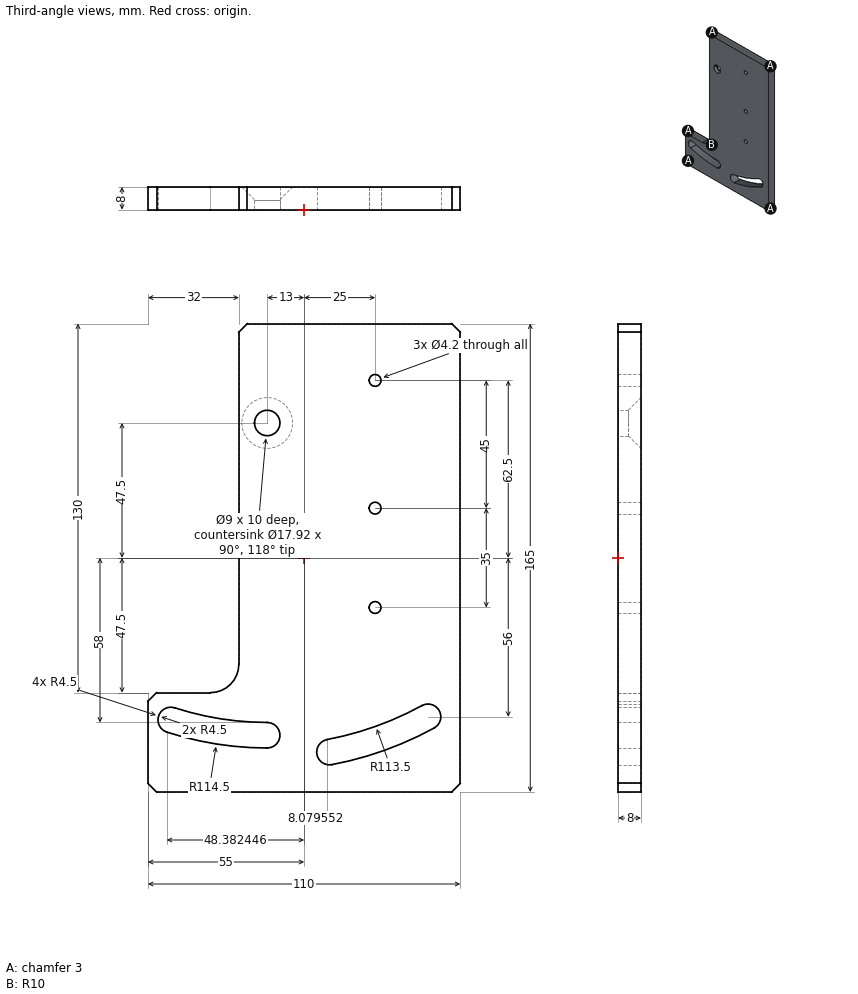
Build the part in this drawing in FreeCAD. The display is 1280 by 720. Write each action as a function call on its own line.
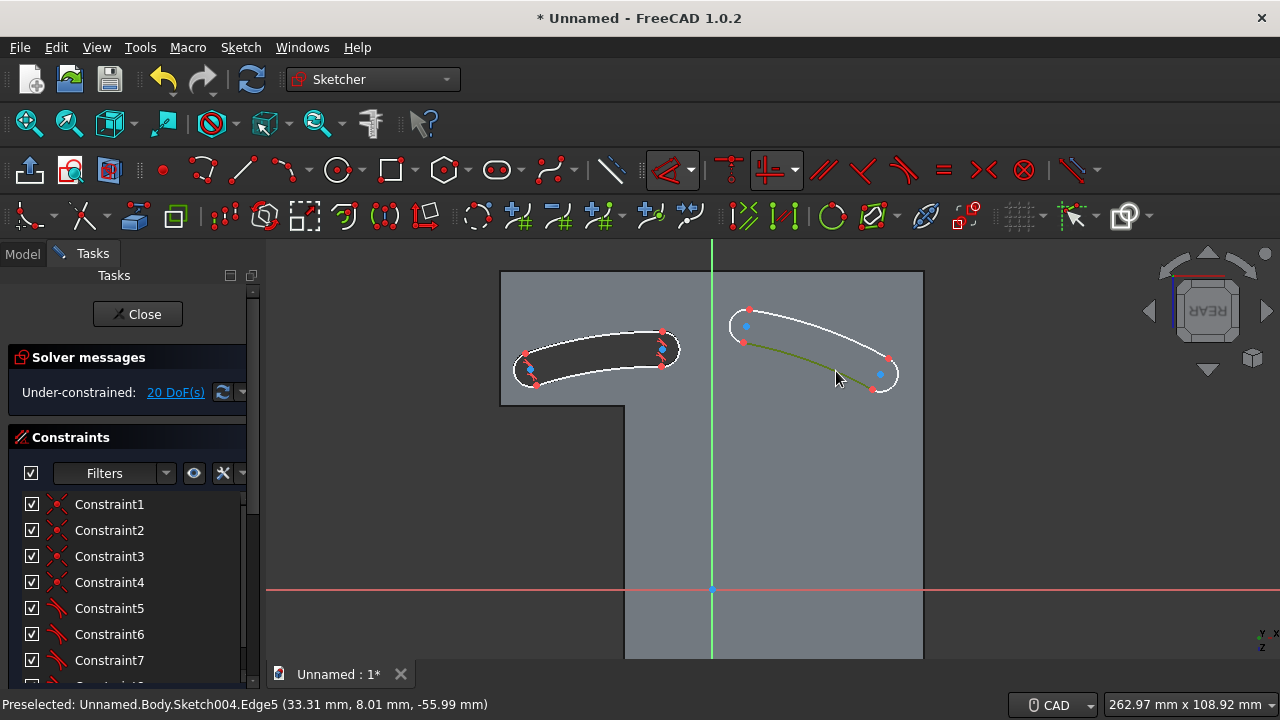
click(888, 390)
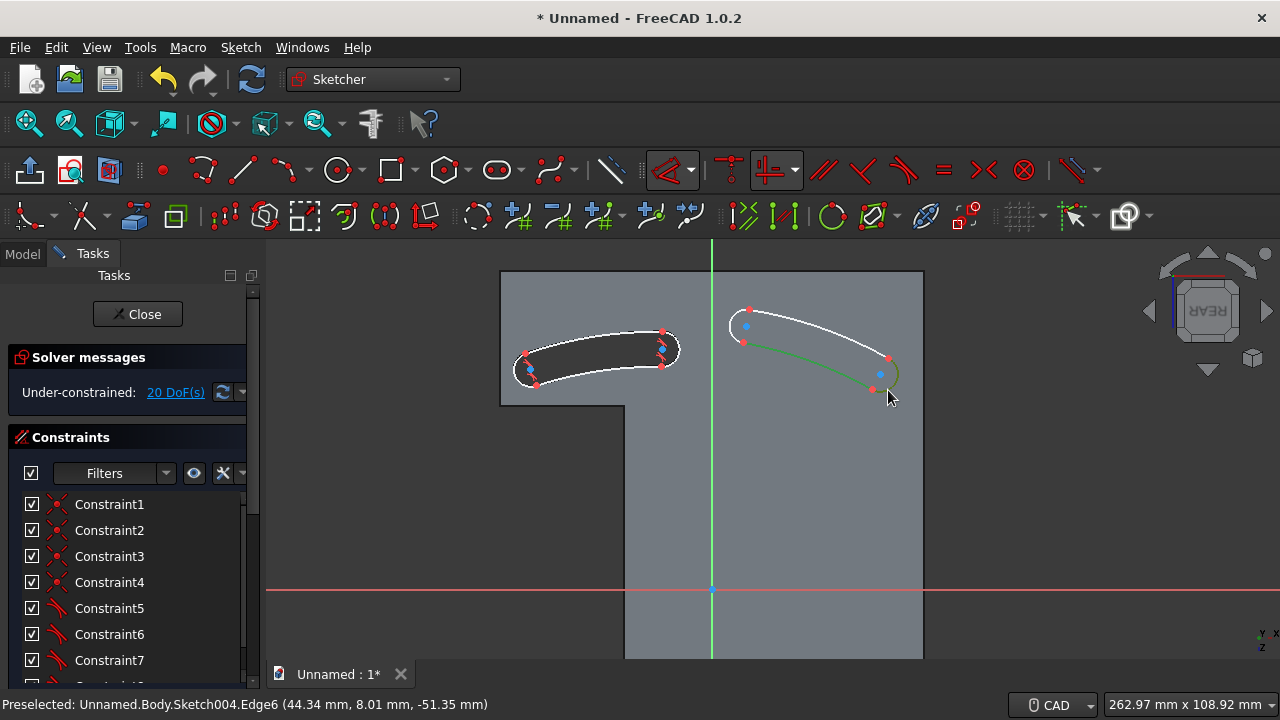
click(904, 170)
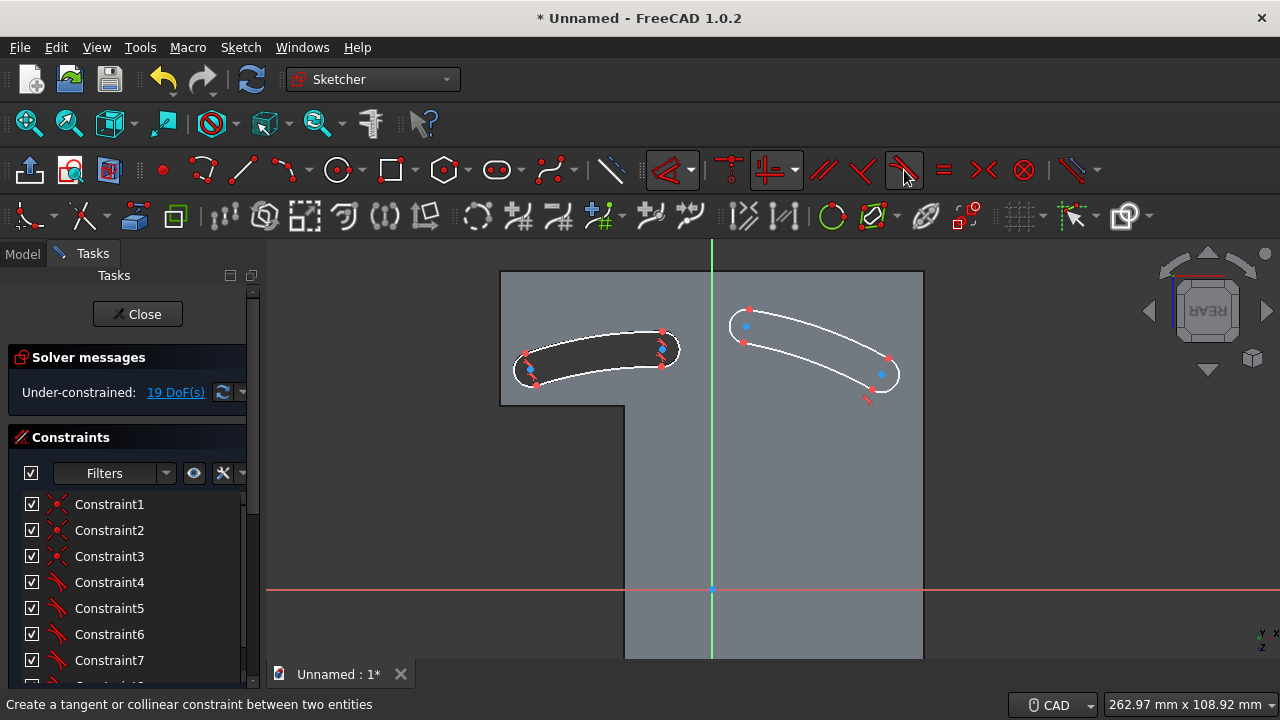
click(836, 371)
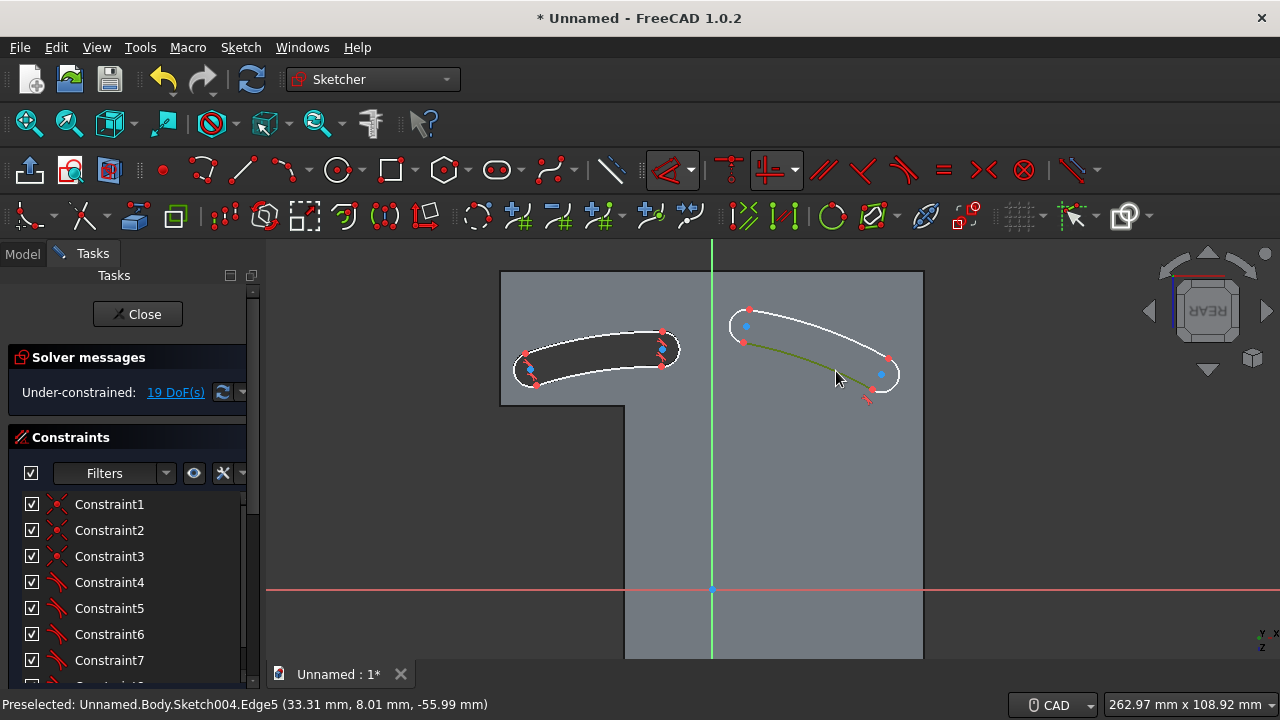
click(735, 314)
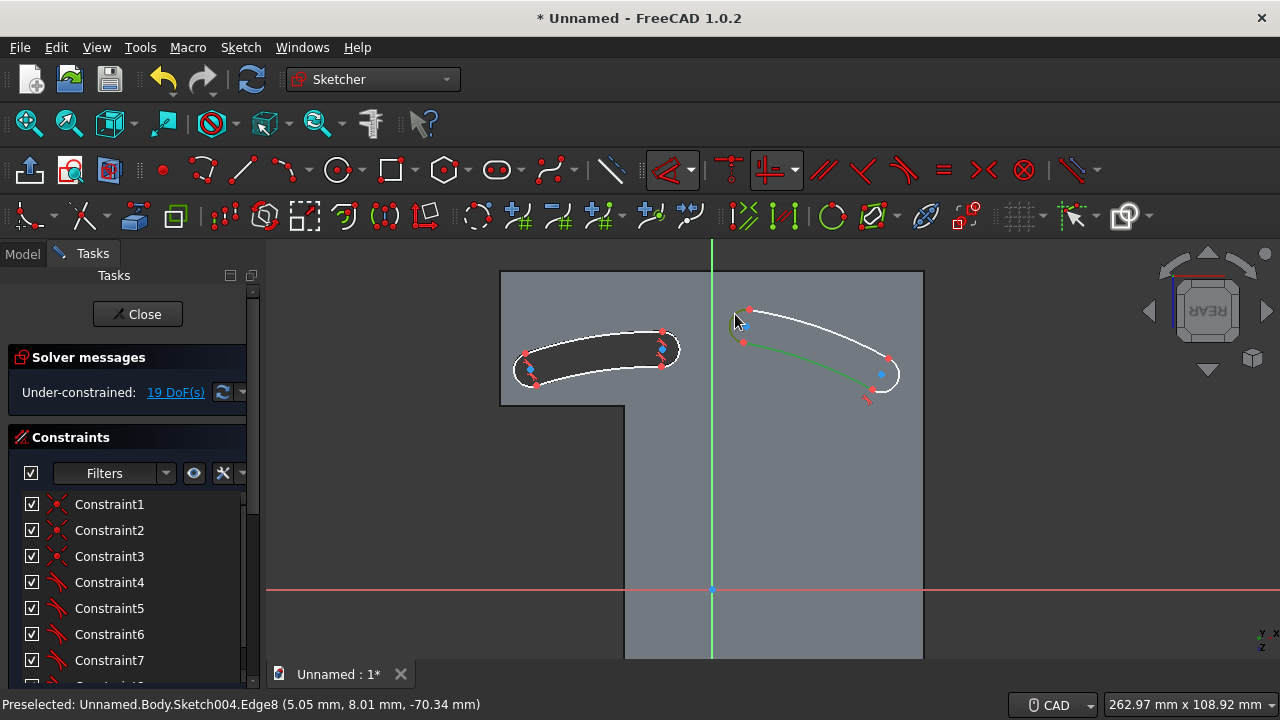
click(904, 170)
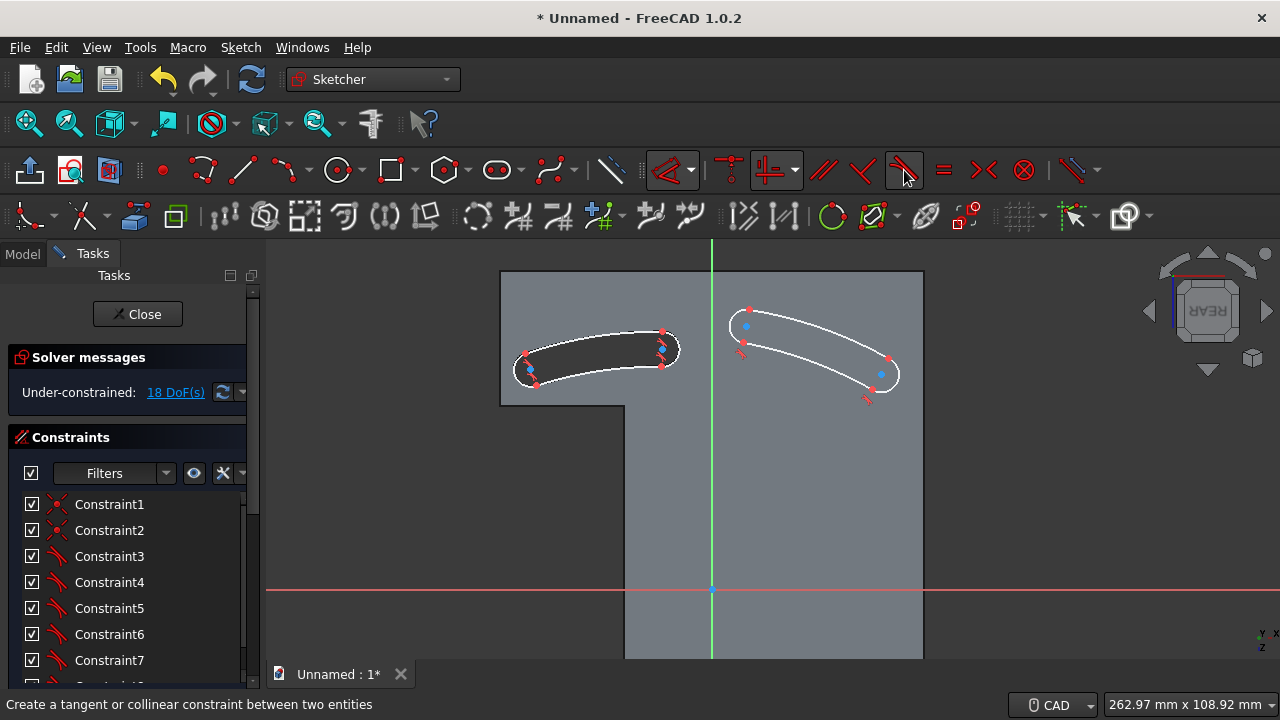
click(889, 391)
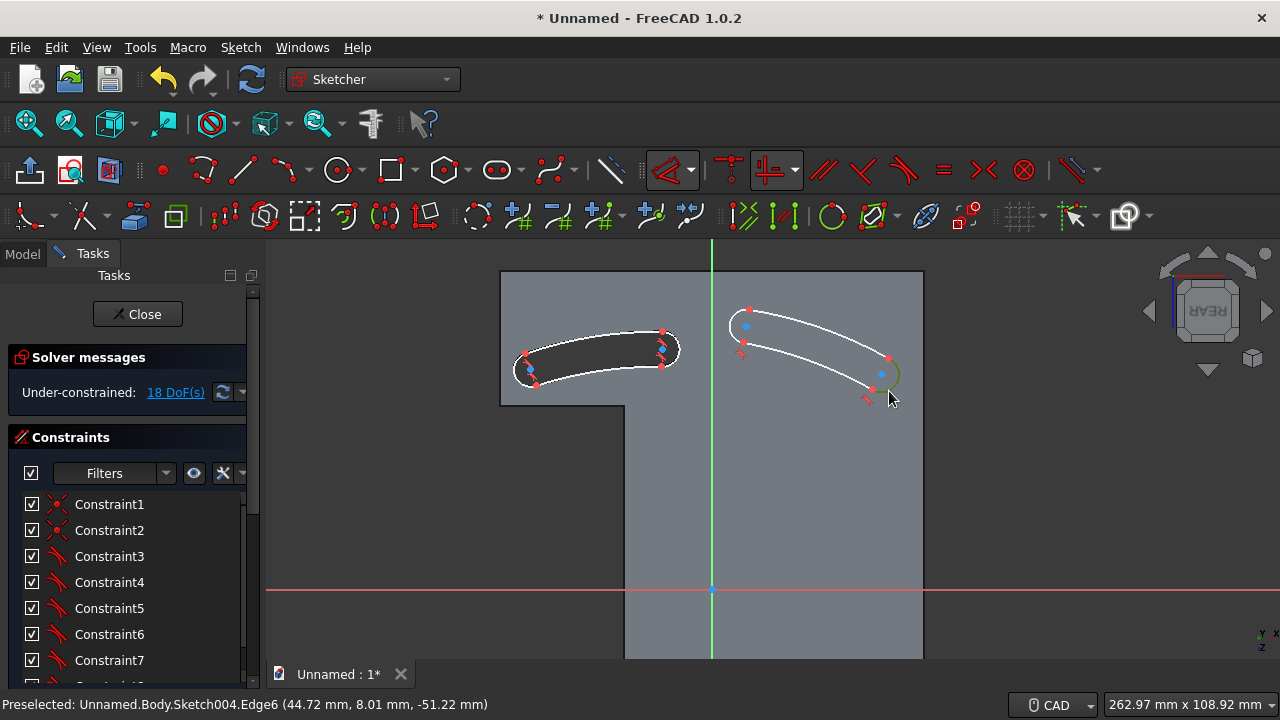
click(849, 339)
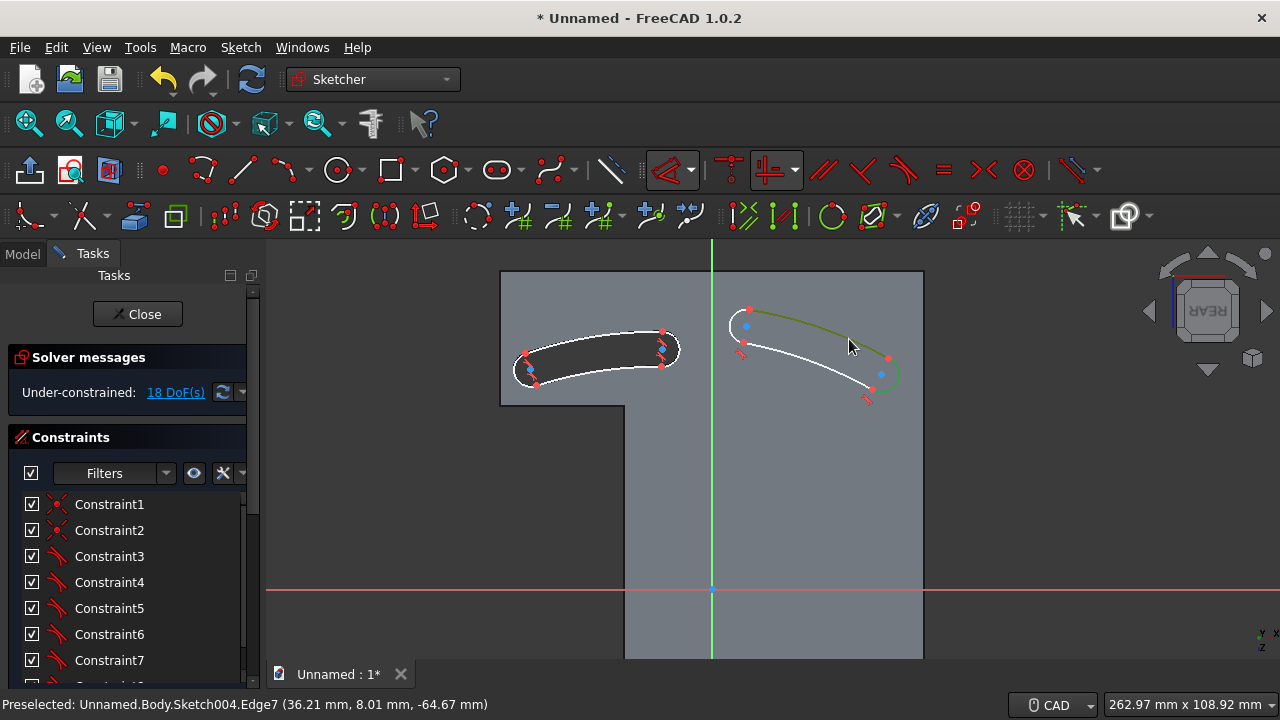
click(904, 170)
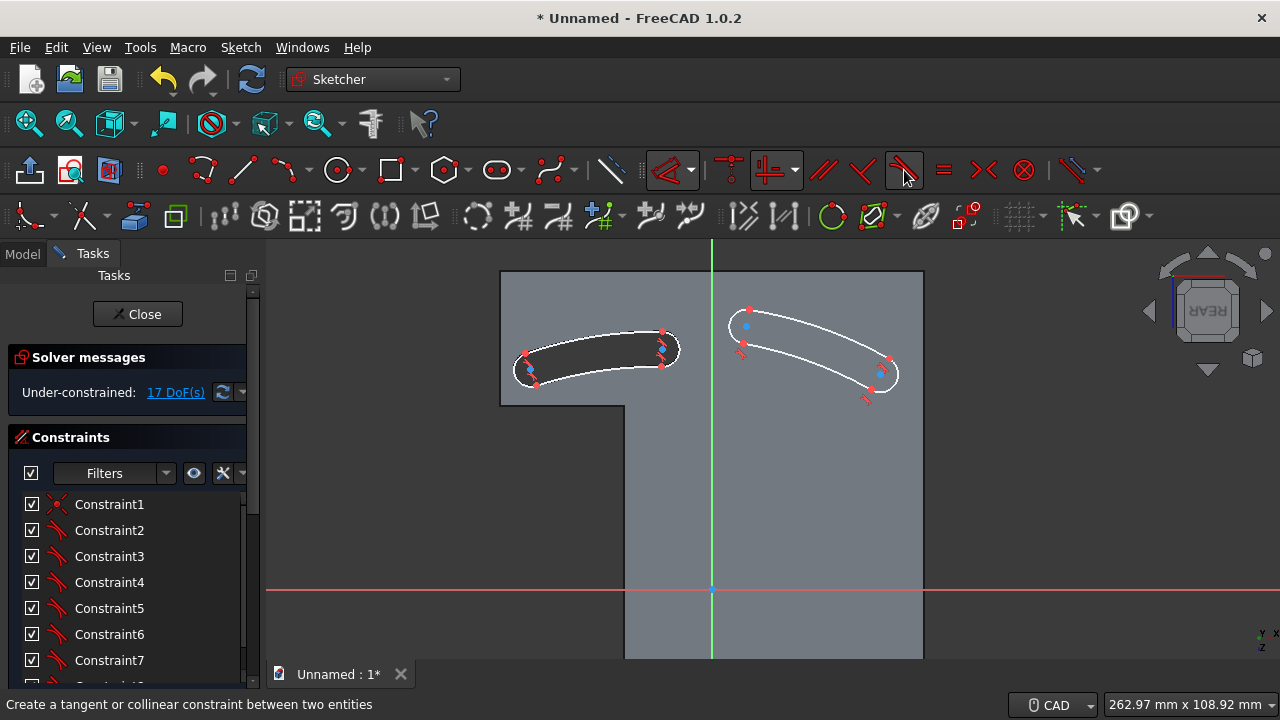
click(849, 339)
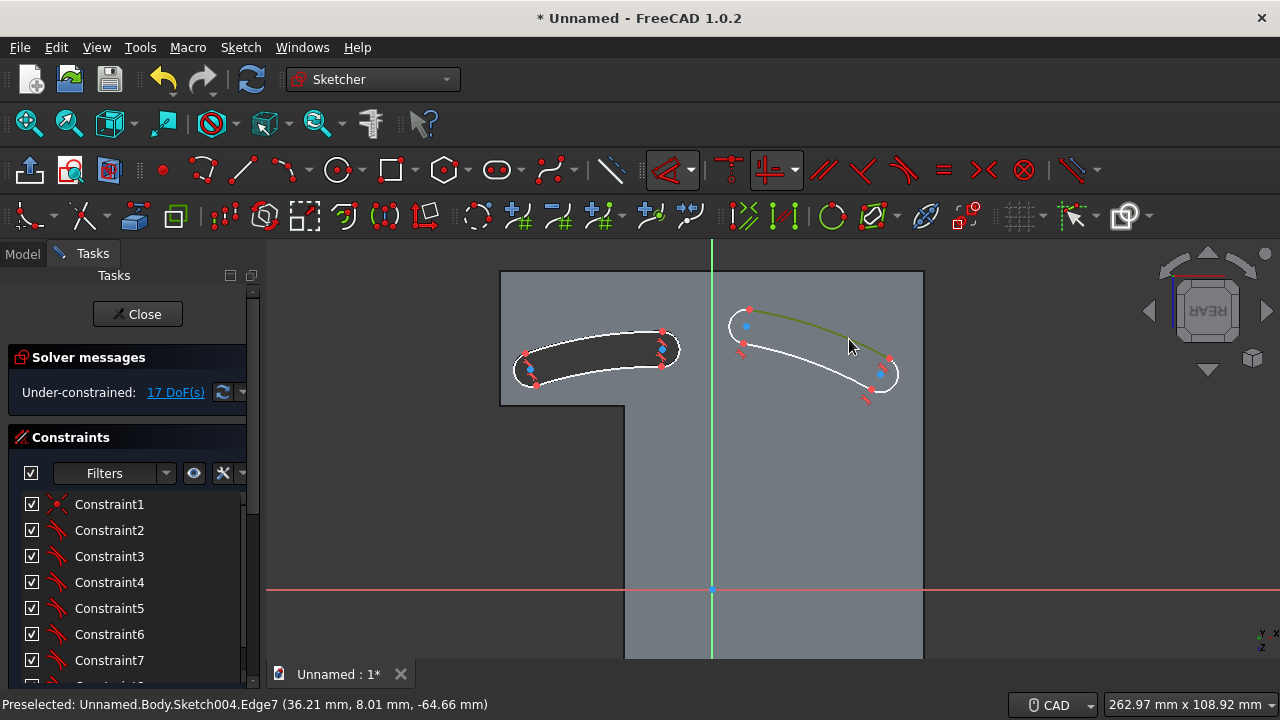
click(735, 314)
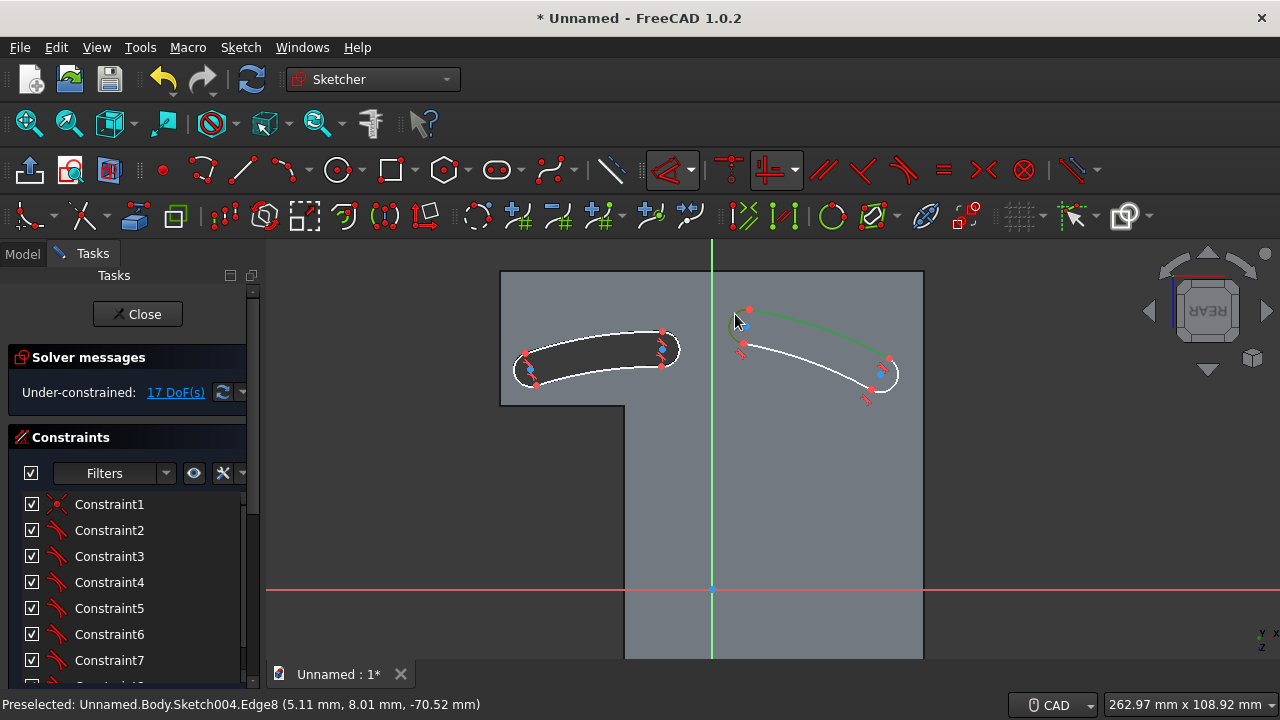
click(904, 170)